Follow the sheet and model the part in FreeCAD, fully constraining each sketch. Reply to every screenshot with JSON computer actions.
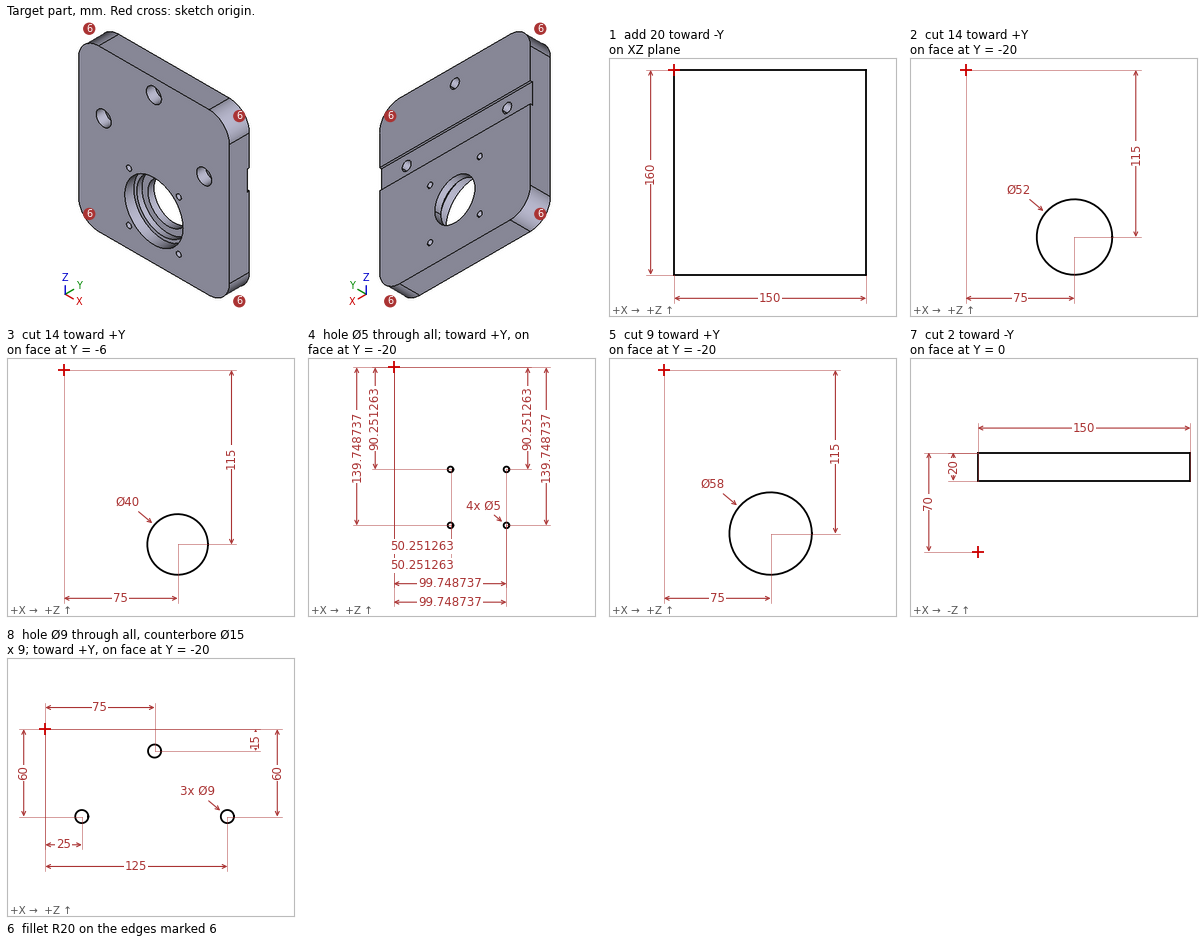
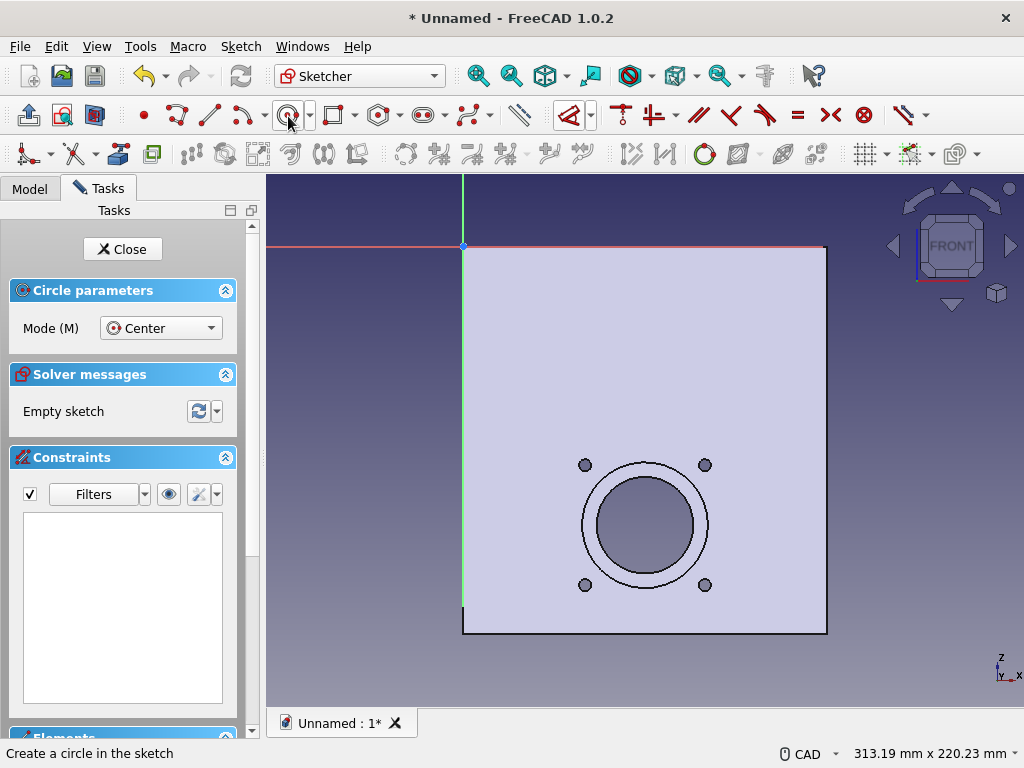
{"action": "left_click", "coordinate": [645, 525]}
{"action": "left_click", "coordinate": [695, 476]}
{"action": "key", "text": "Escape"}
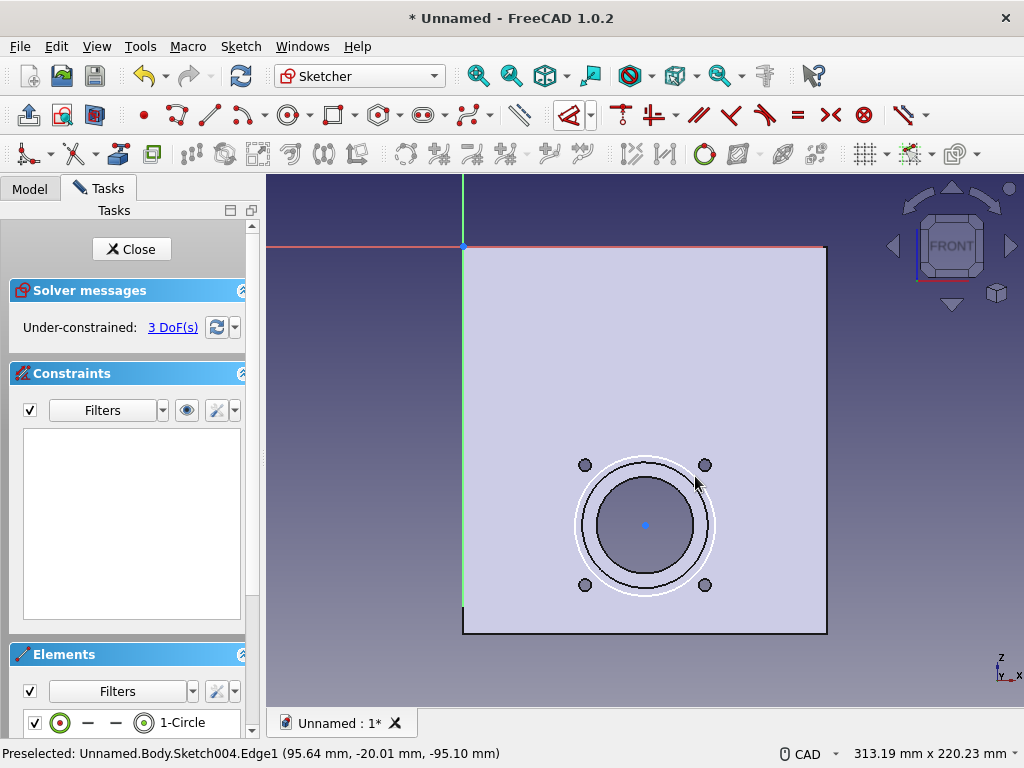
{"action": "left_click", "coordinate": [694, 476]}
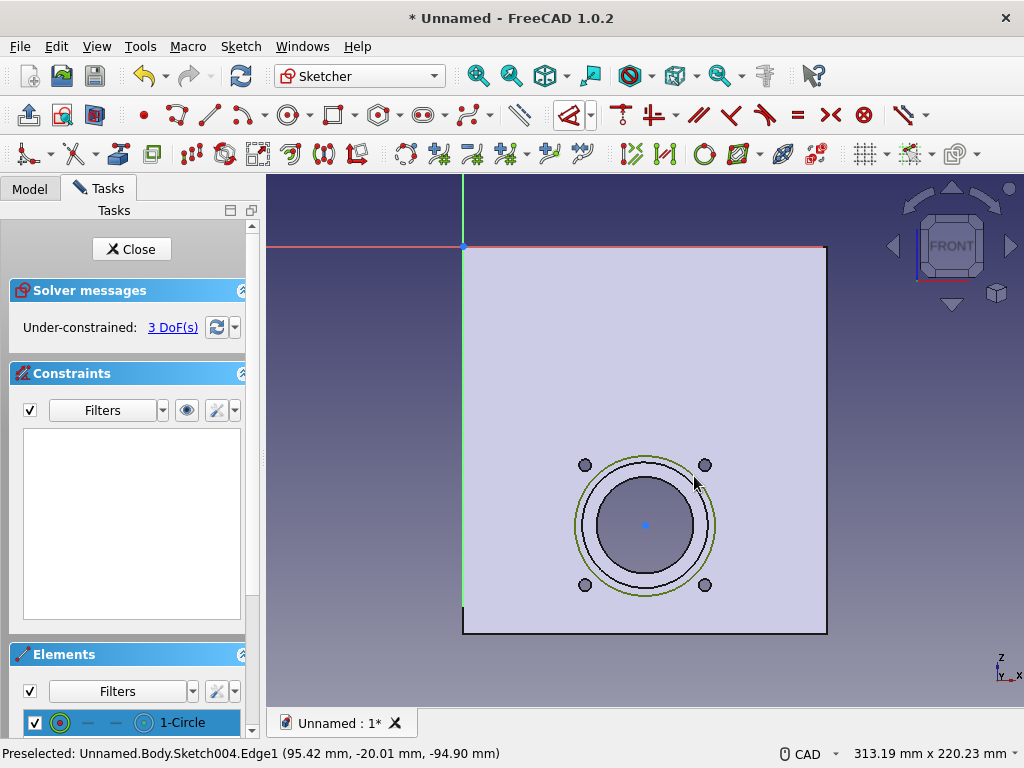
{"action": "left_click", "coordinate": [590, 116]}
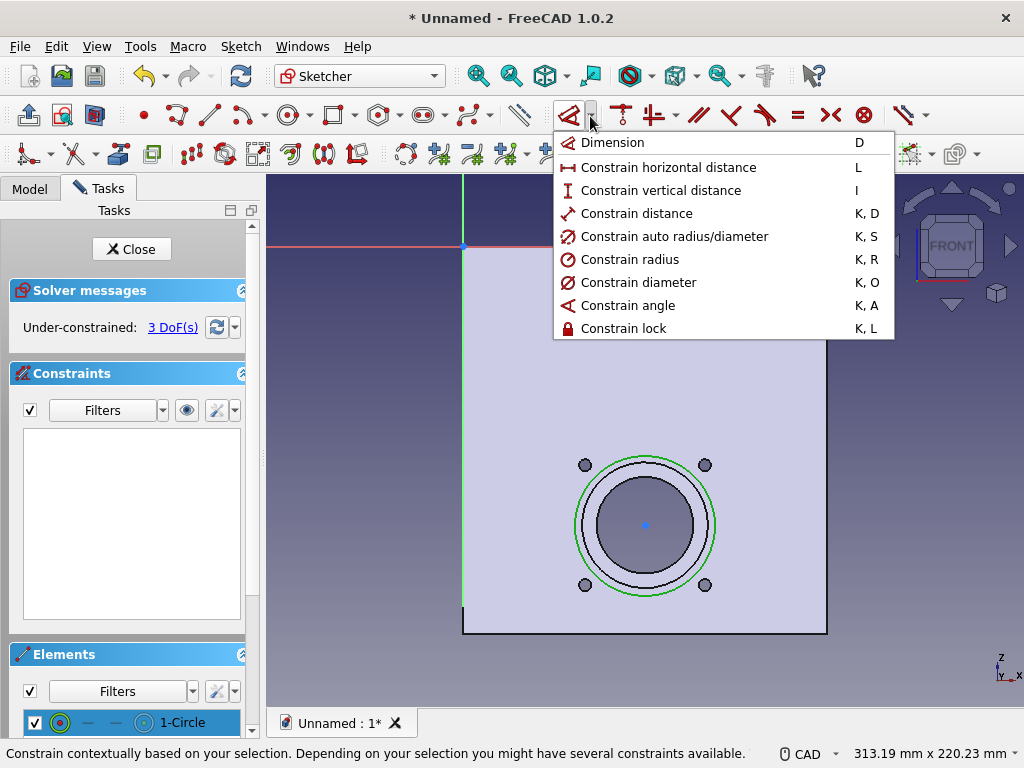
{"action": "left_click", "coordinate": [724, 282]}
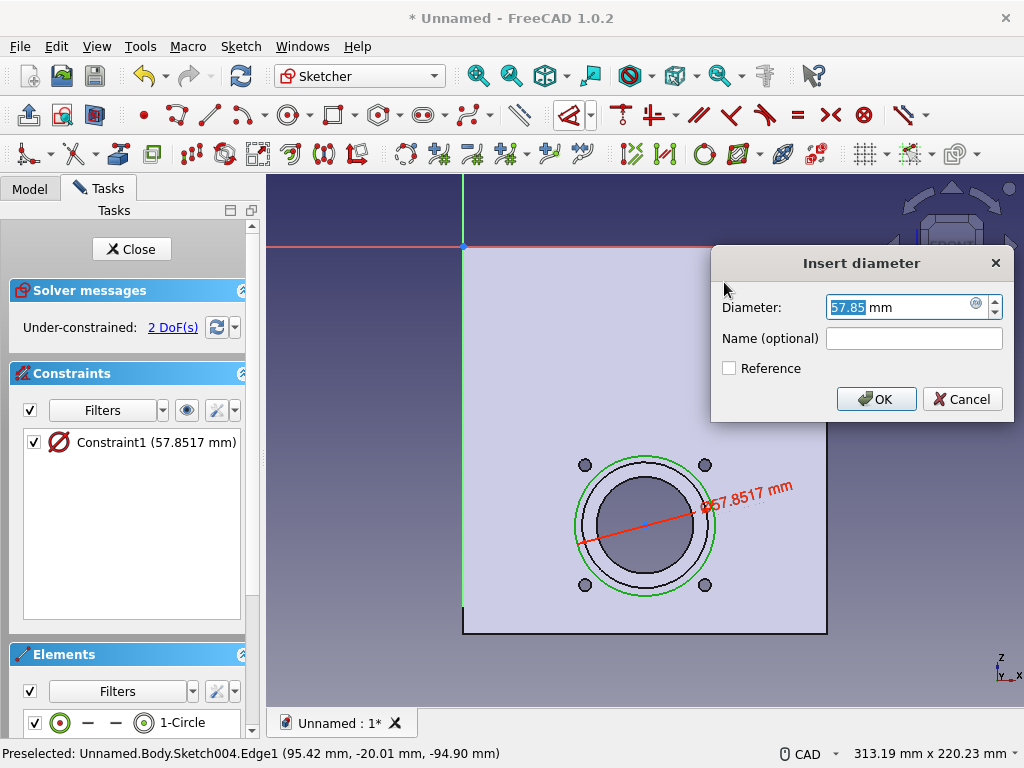
{"action": "type", "text": "58"}
{"action": "key", "text": "Return"}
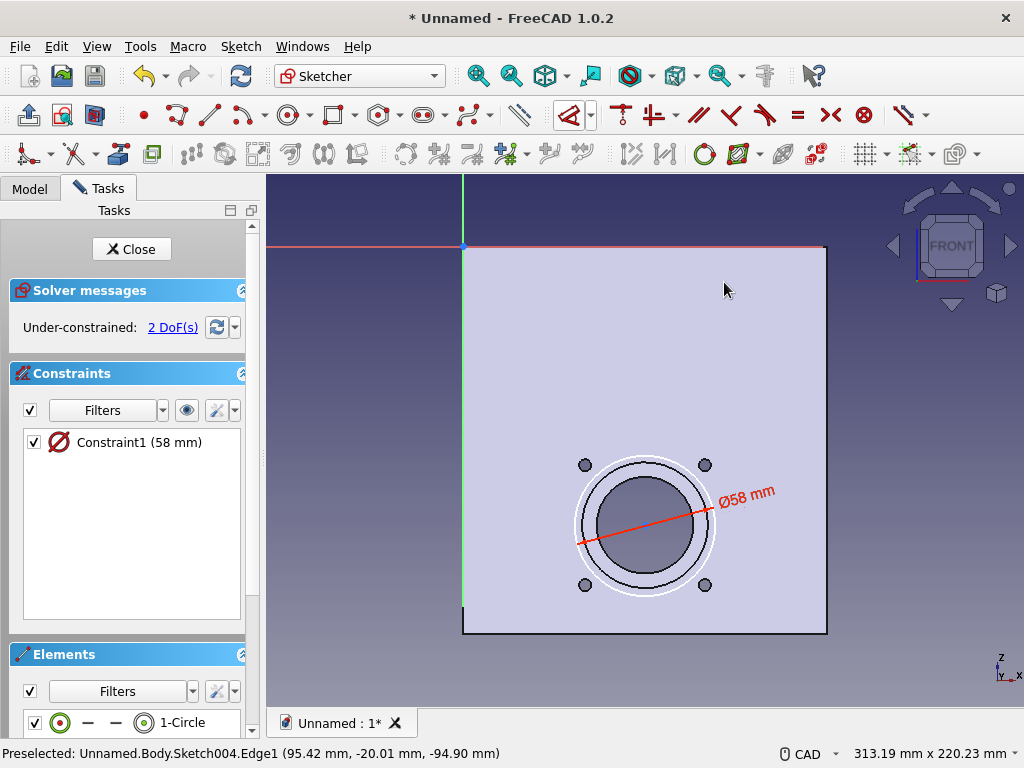
{"action": "left_click", "coordinate": [645, 526]}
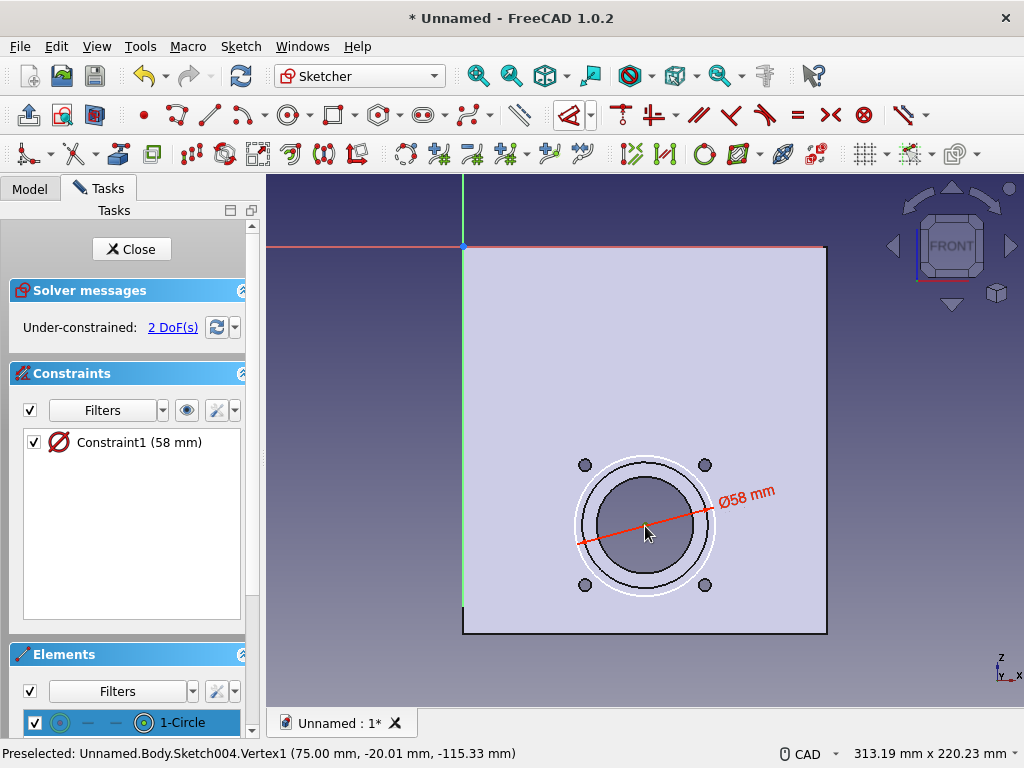
{"action": "key", "text": "l"}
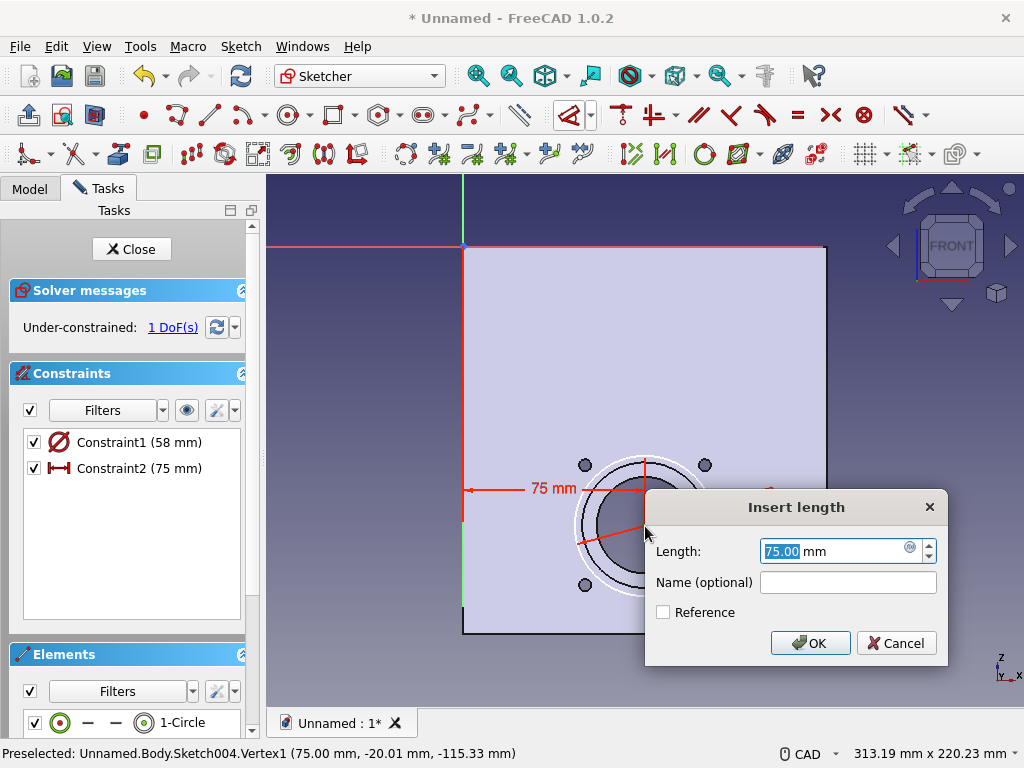
{"action": "type", "text": "75"}
{"action": "key", "text": "Return"}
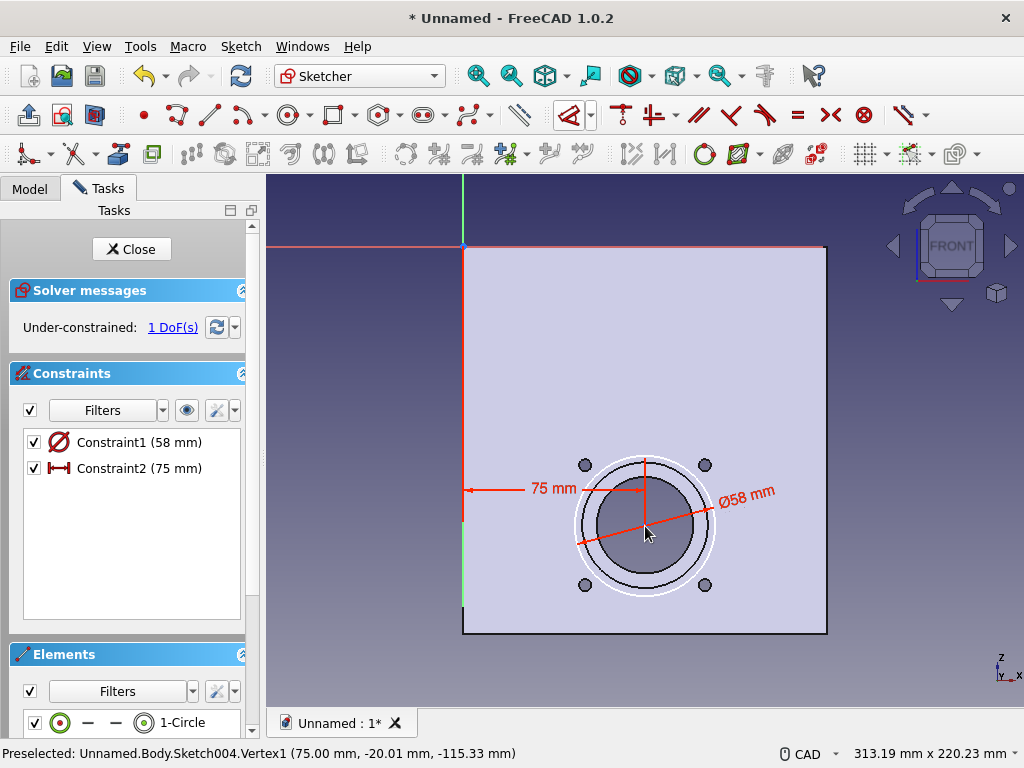
{"action": "left_click", "coordinate": [645, 526]}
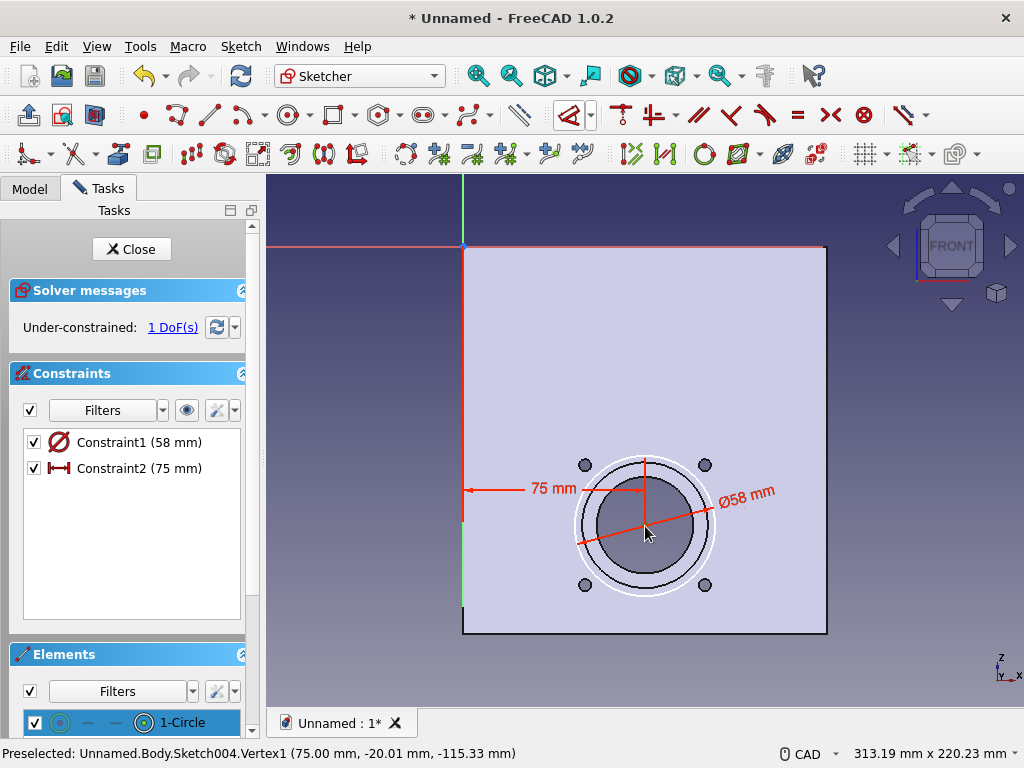
{"action": "key", "text": "i"}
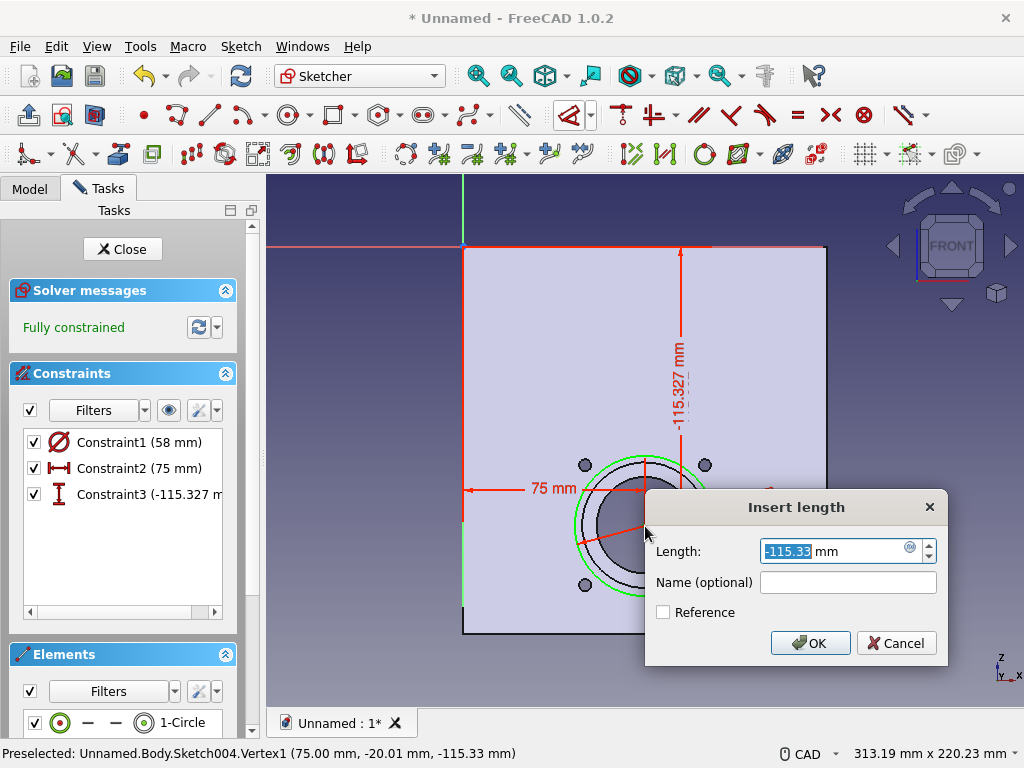
{"action": "type", "text": "-115"}
{"action": "key", "text": "Return"}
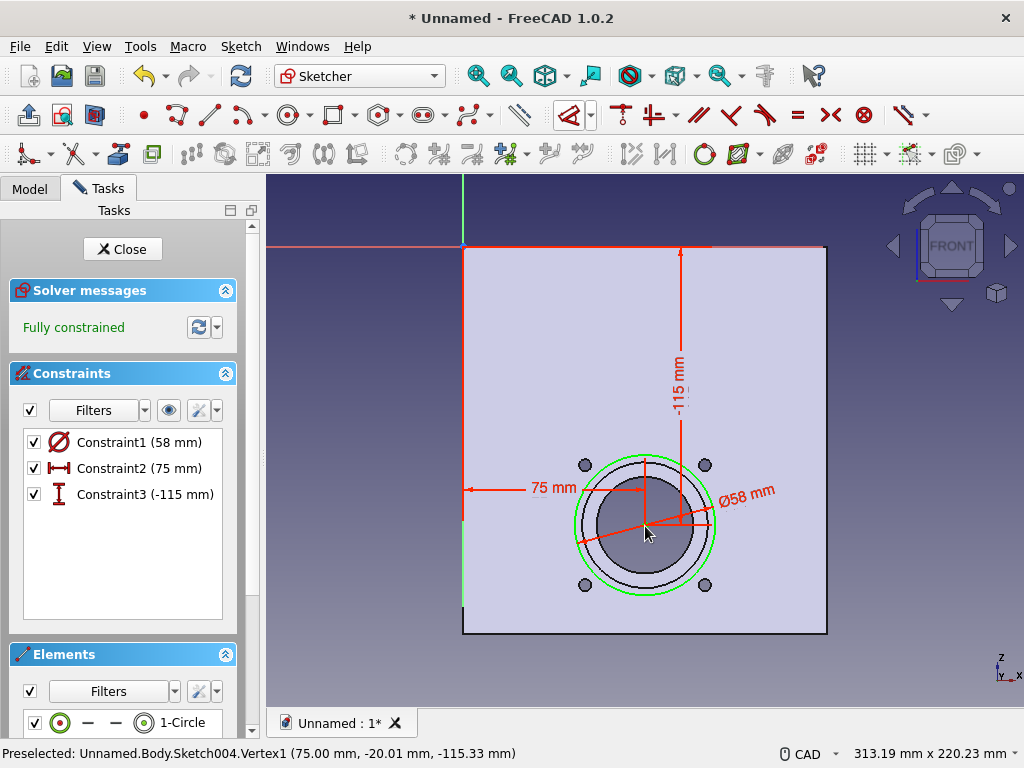
{"action": "left_click", "coordinate": [123, 249]}